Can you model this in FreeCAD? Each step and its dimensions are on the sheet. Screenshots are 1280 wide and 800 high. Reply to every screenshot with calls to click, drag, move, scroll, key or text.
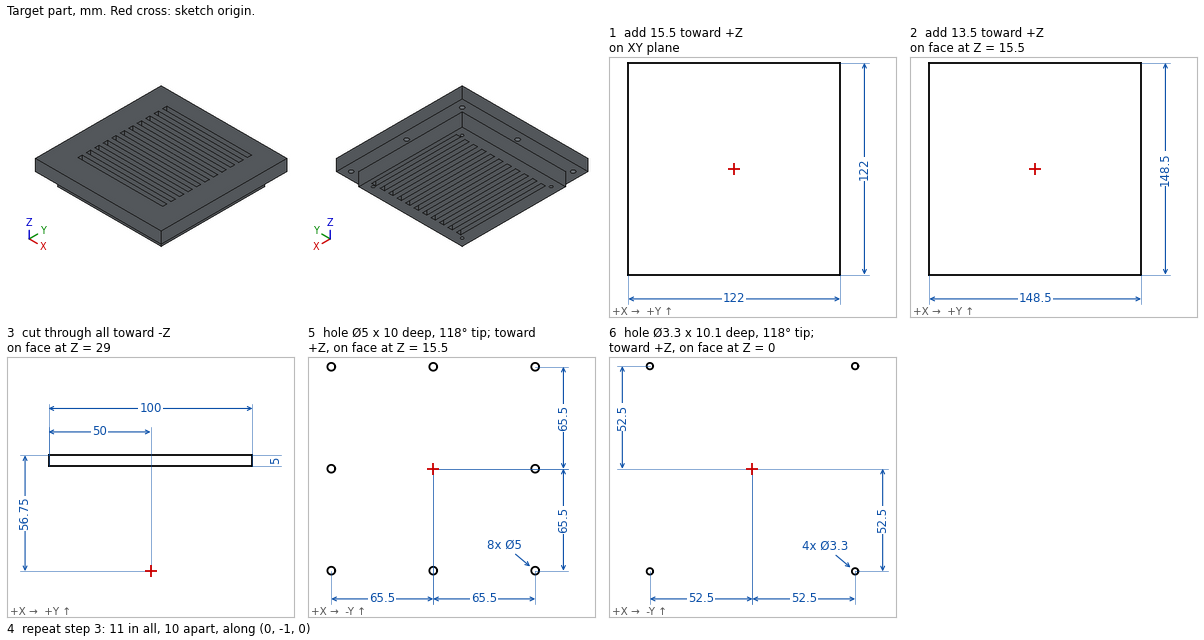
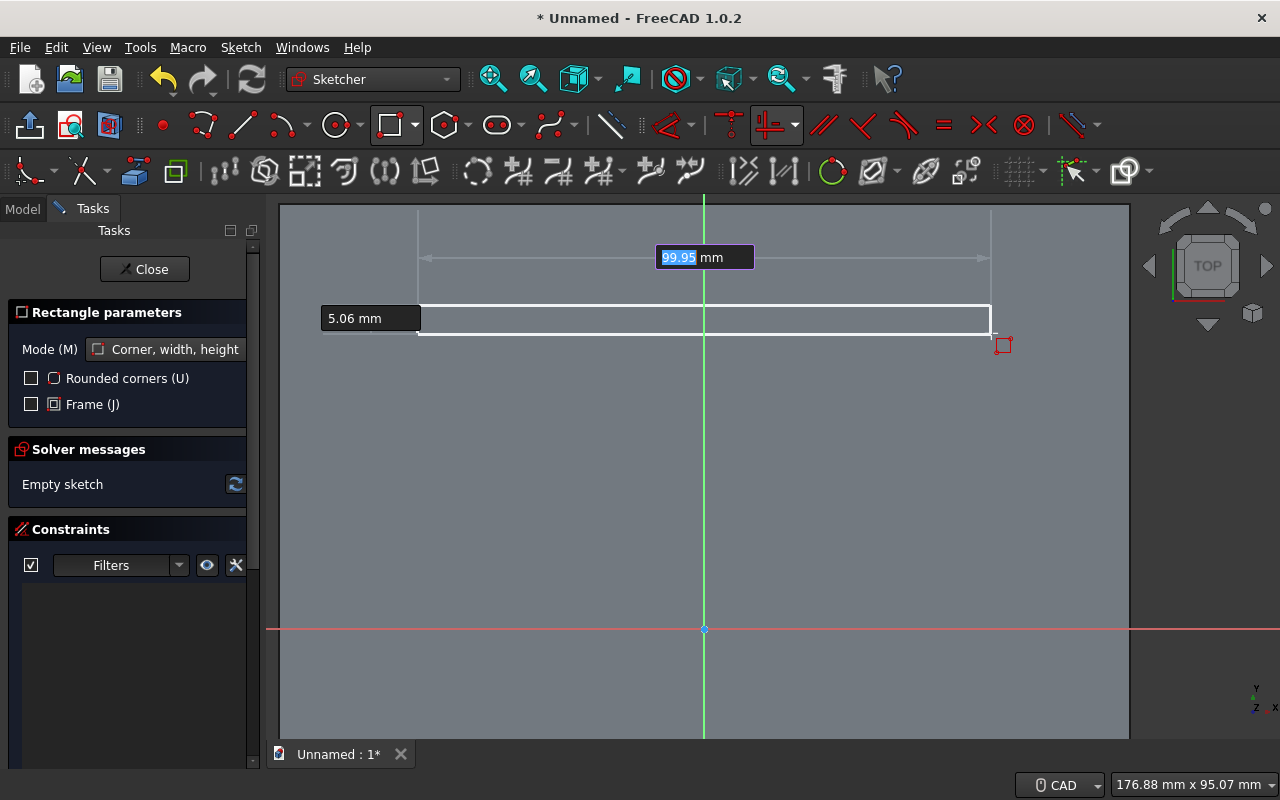
text(100)
key(Tab)
text(5)
key(Return)
key(Escape)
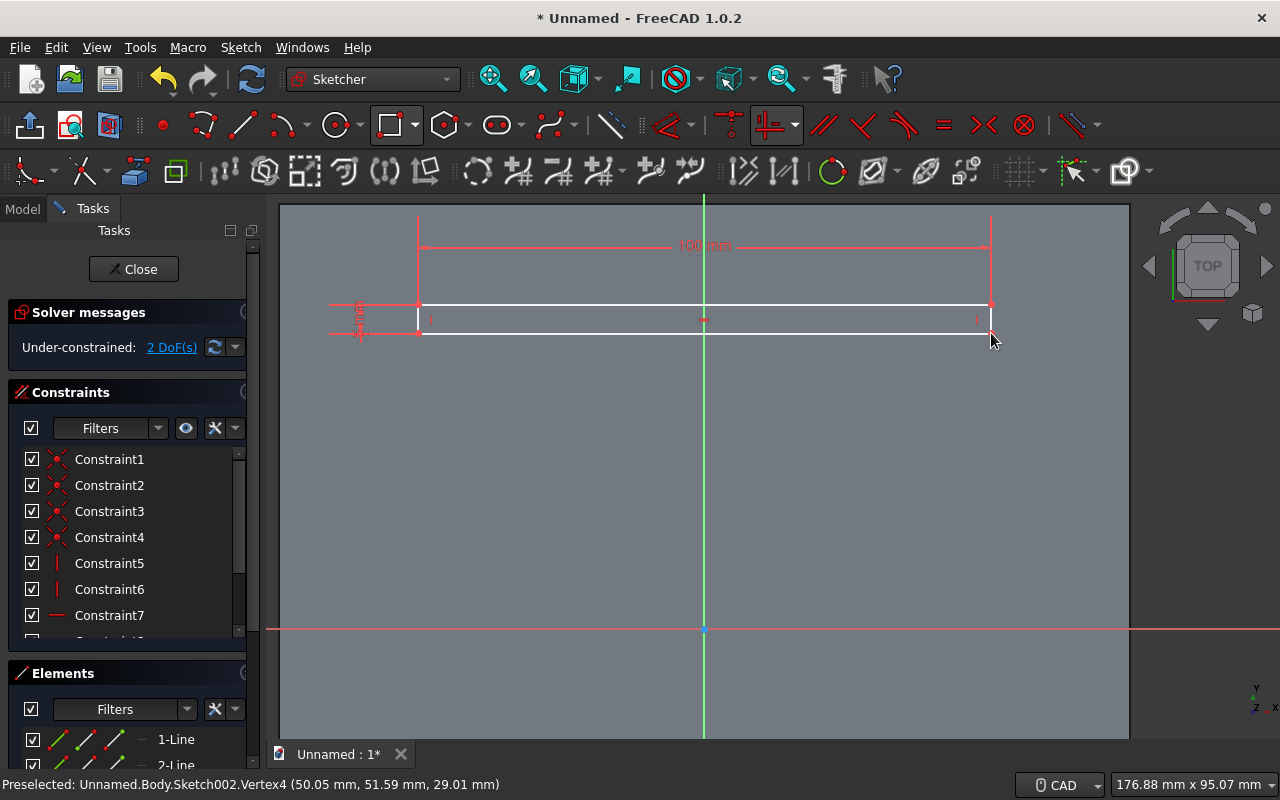
click(418, 305)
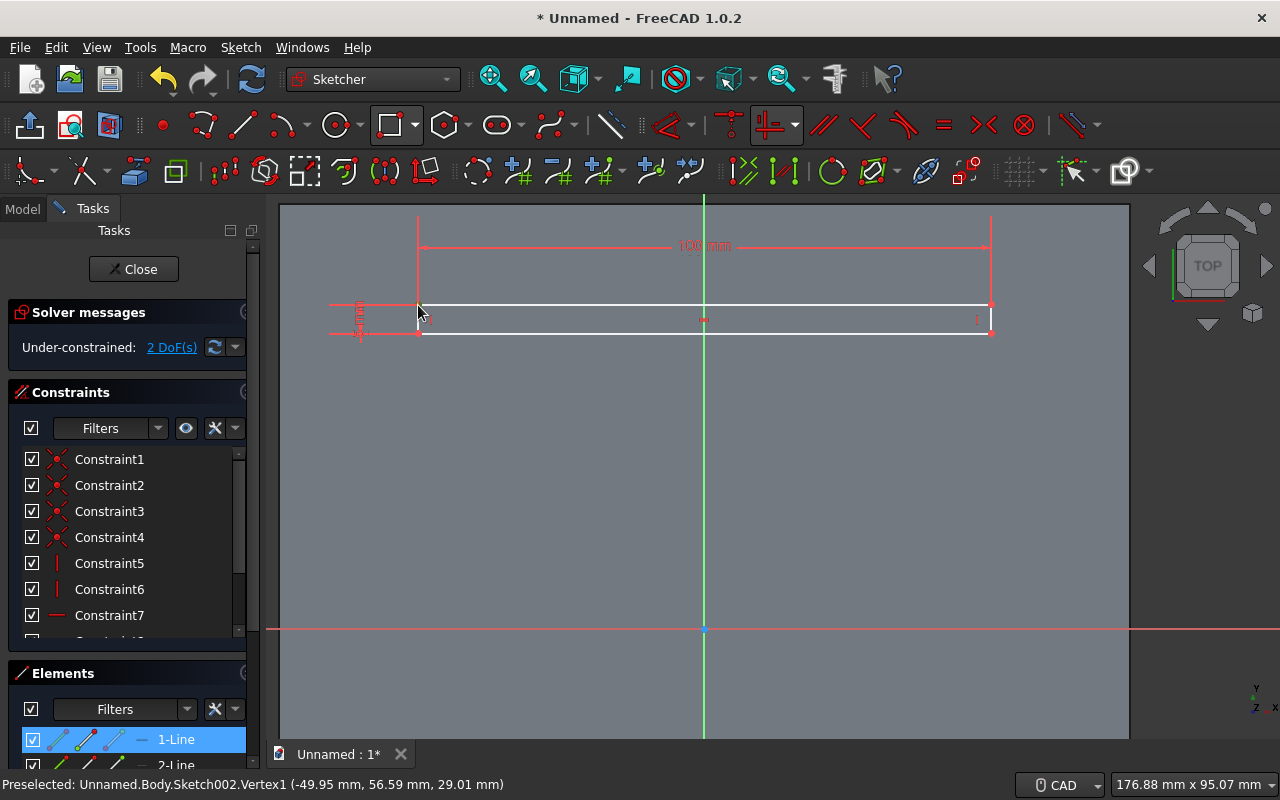
click(694, 126)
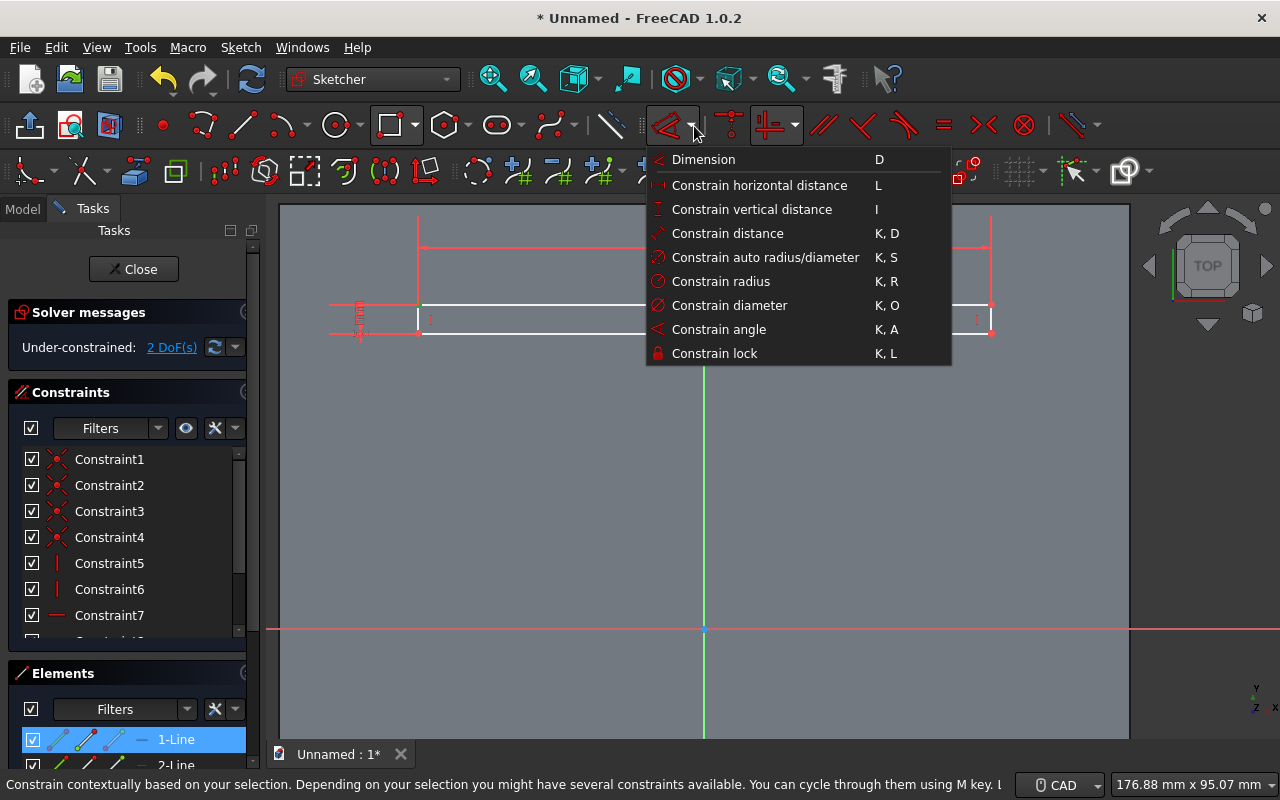
click(799, 185)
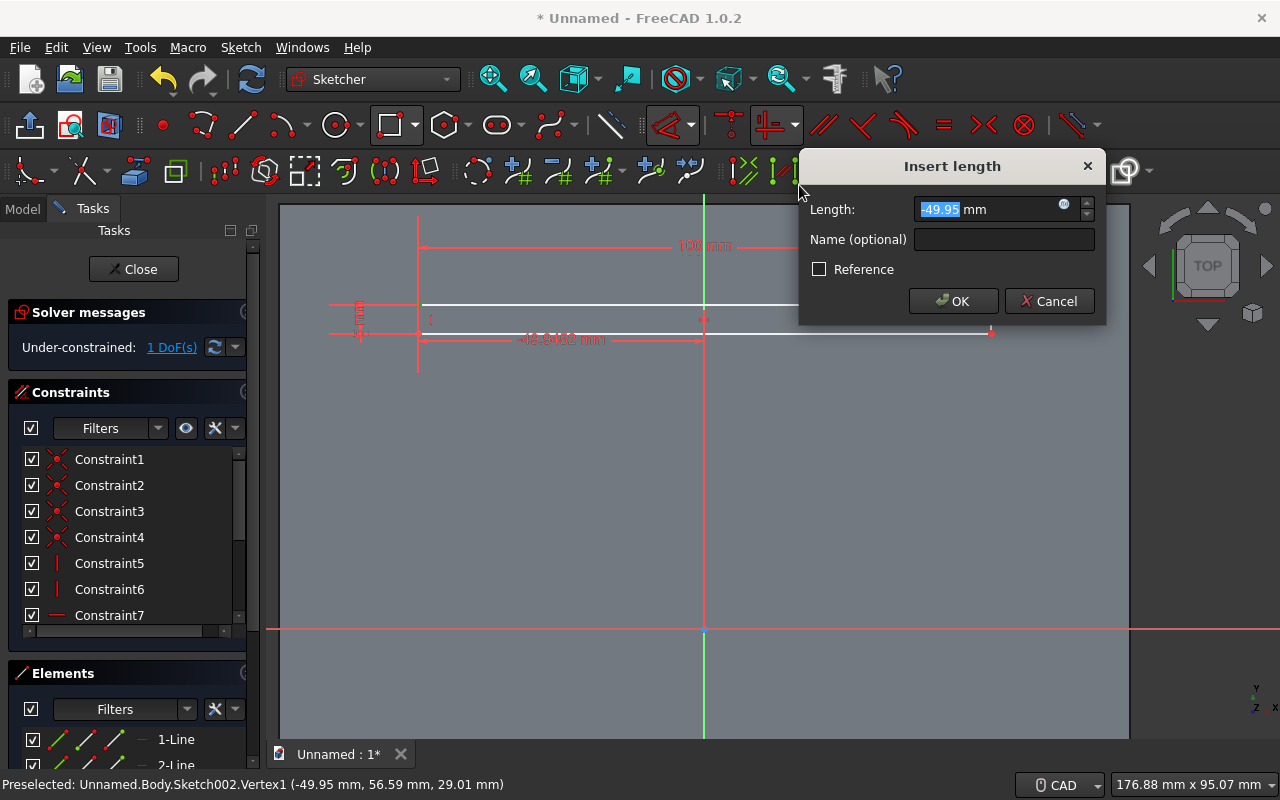
text(-50)
key(Return)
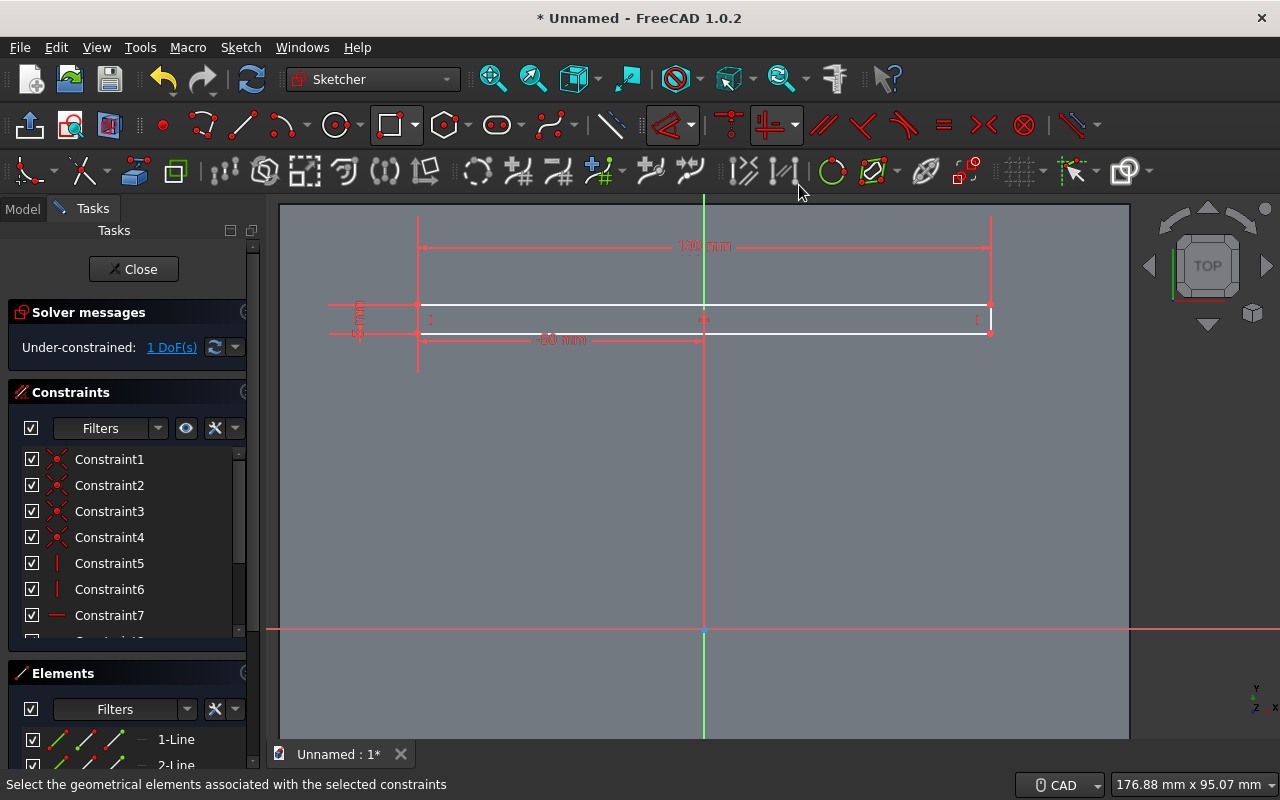
click(418, 305)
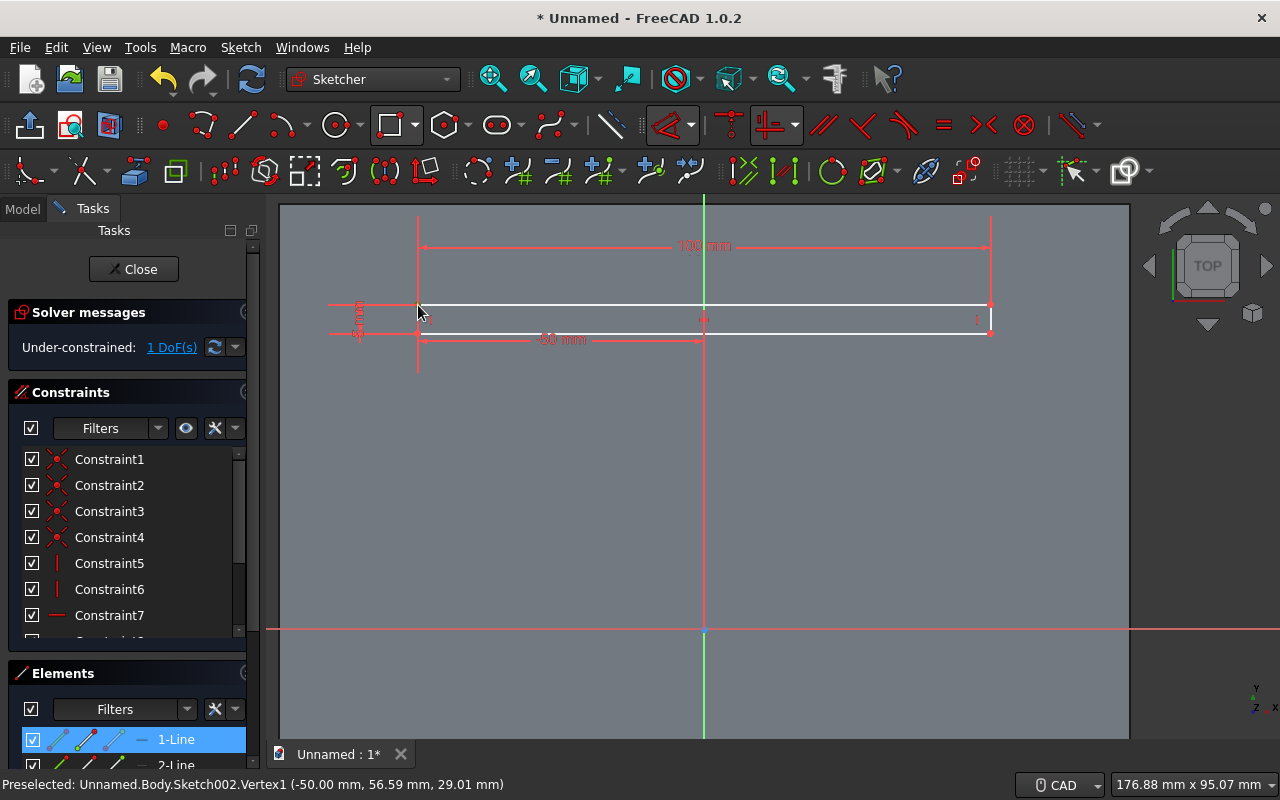
click(694, 126)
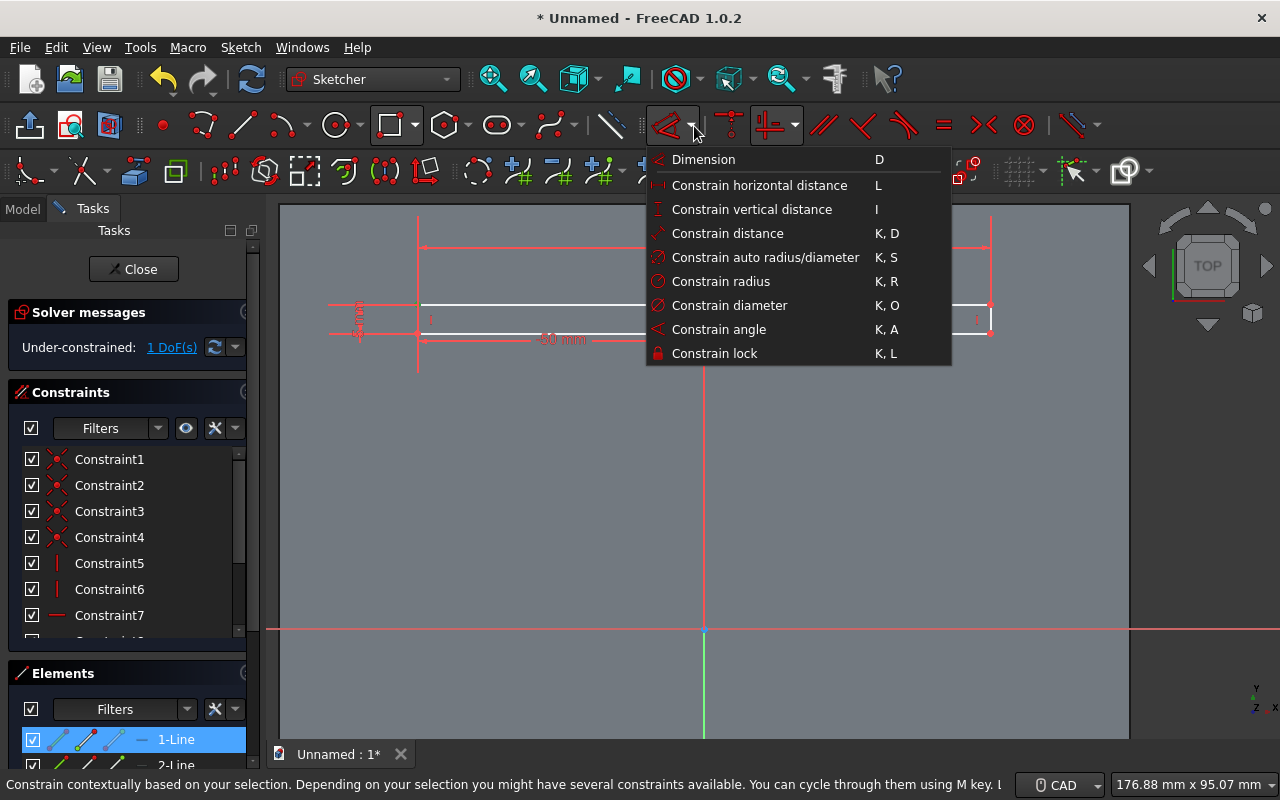
click(799, 209)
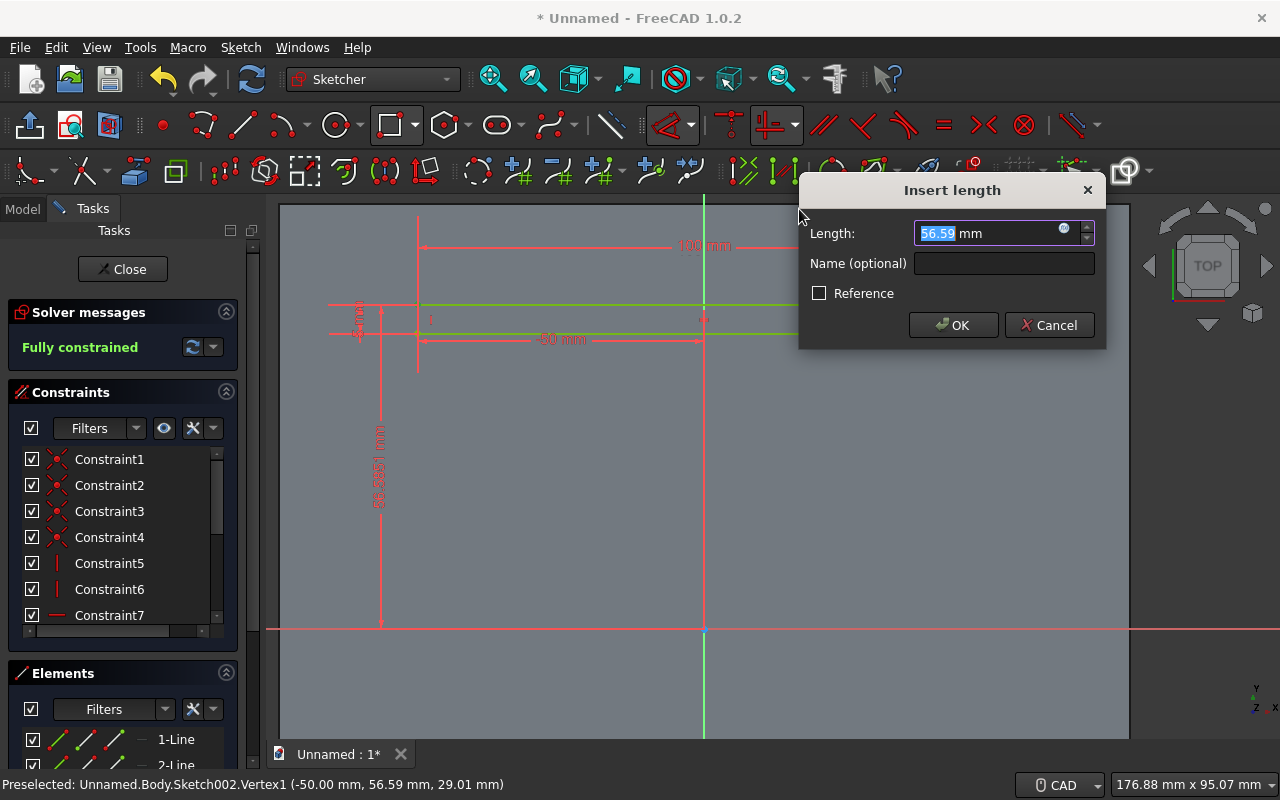
text(56.75)
key(Return)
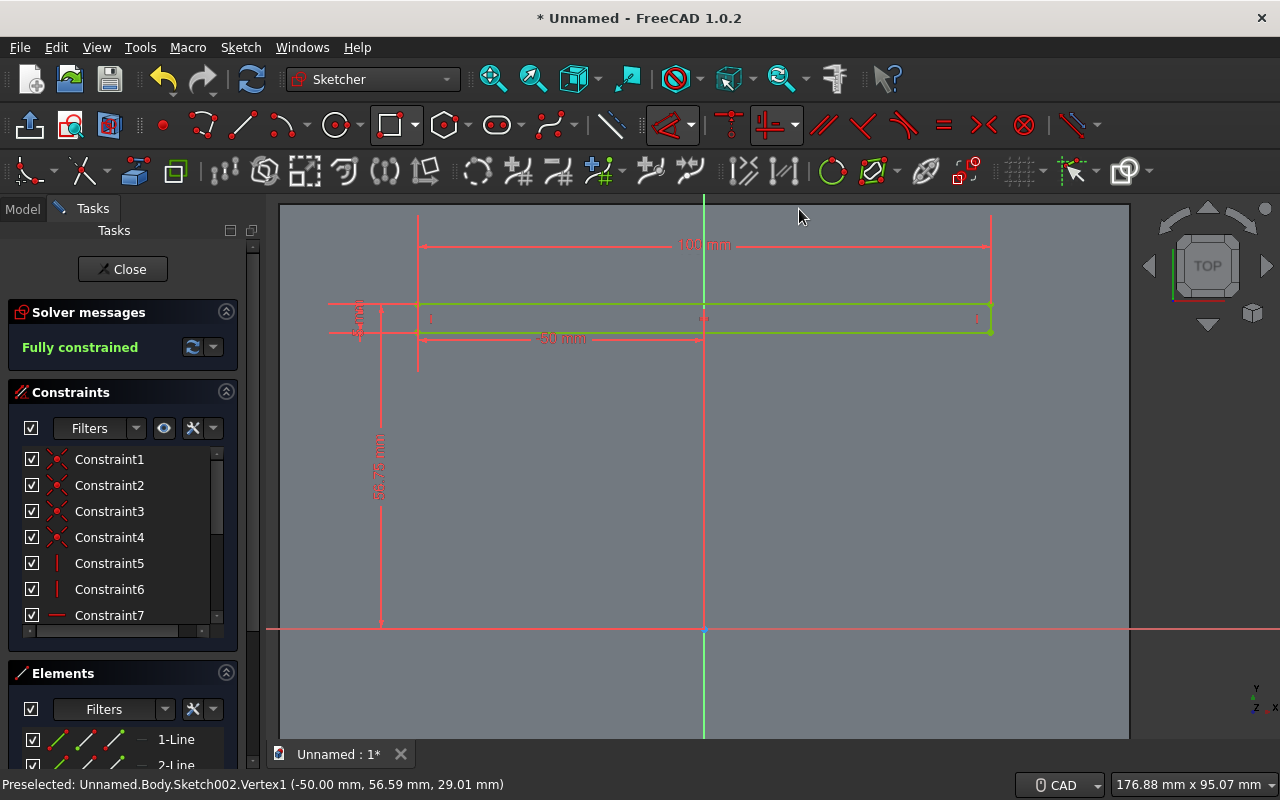
click(123, 269)